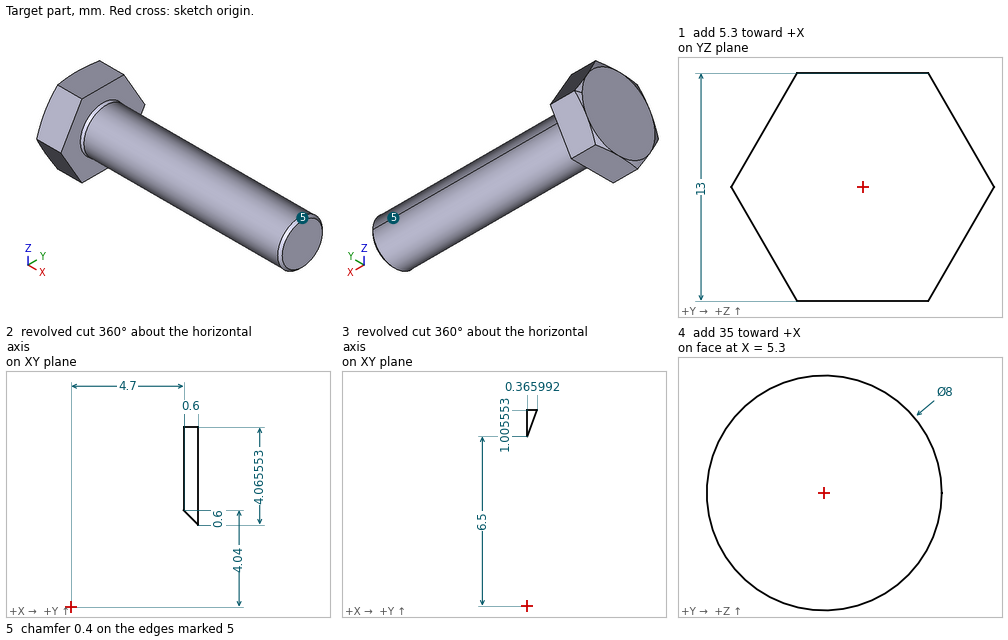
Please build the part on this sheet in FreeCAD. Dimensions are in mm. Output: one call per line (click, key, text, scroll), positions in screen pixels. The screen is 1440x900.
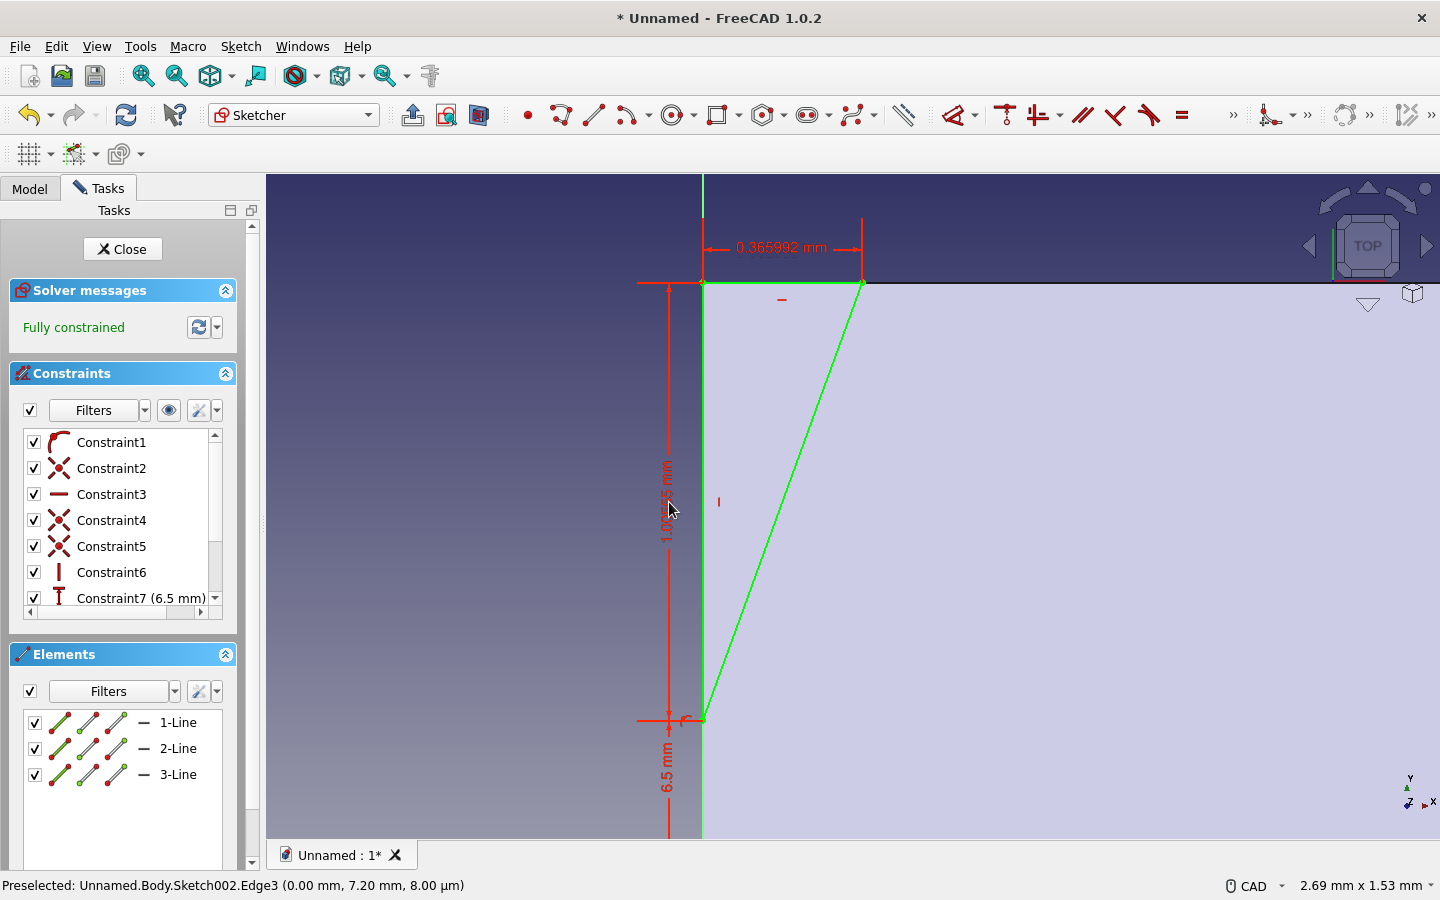
click(123, 249)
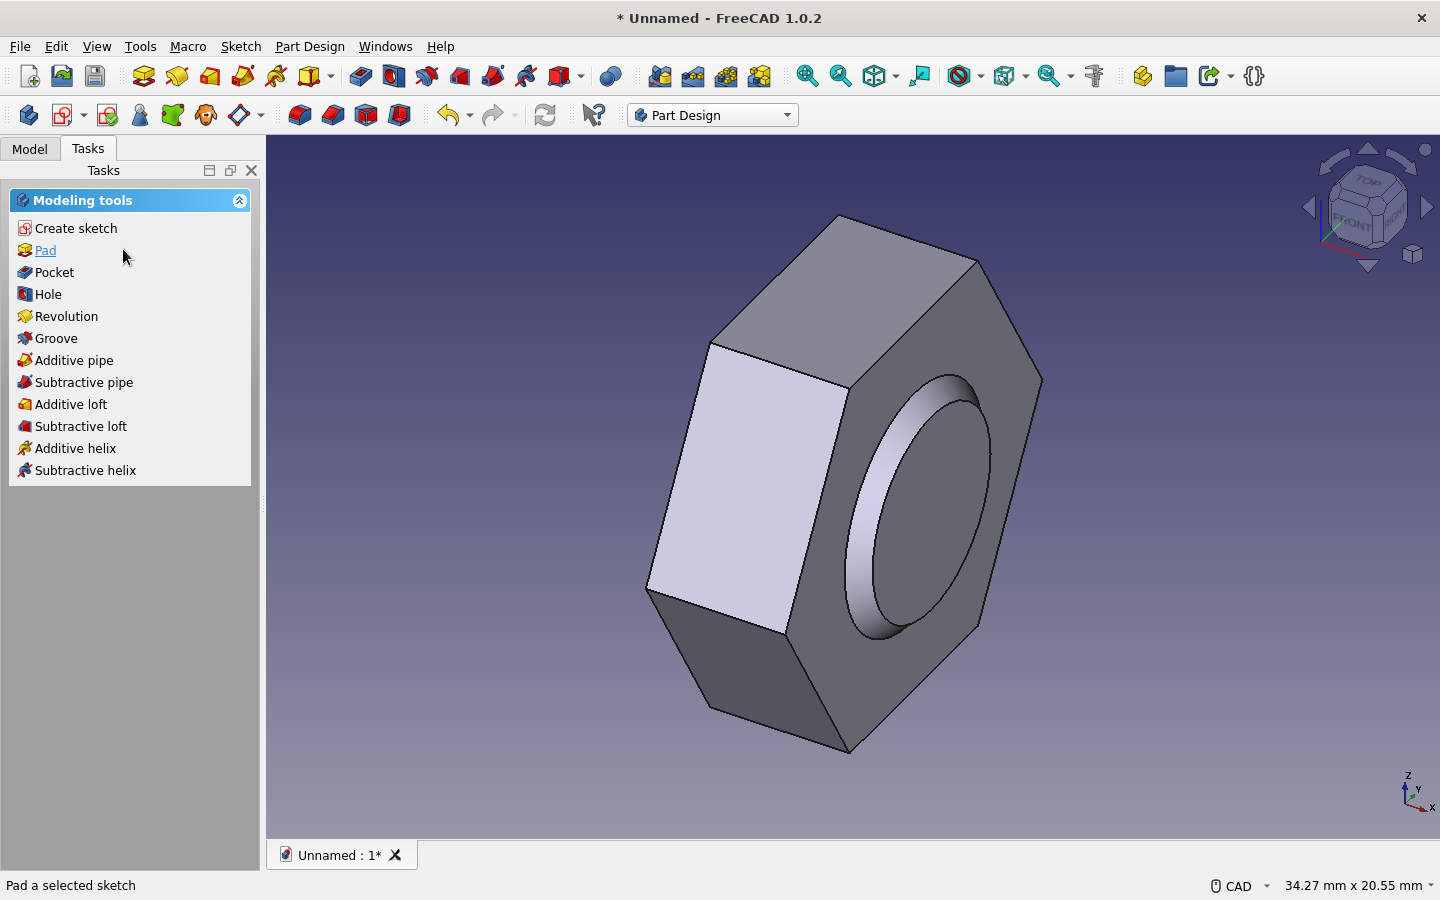
click(427, 76)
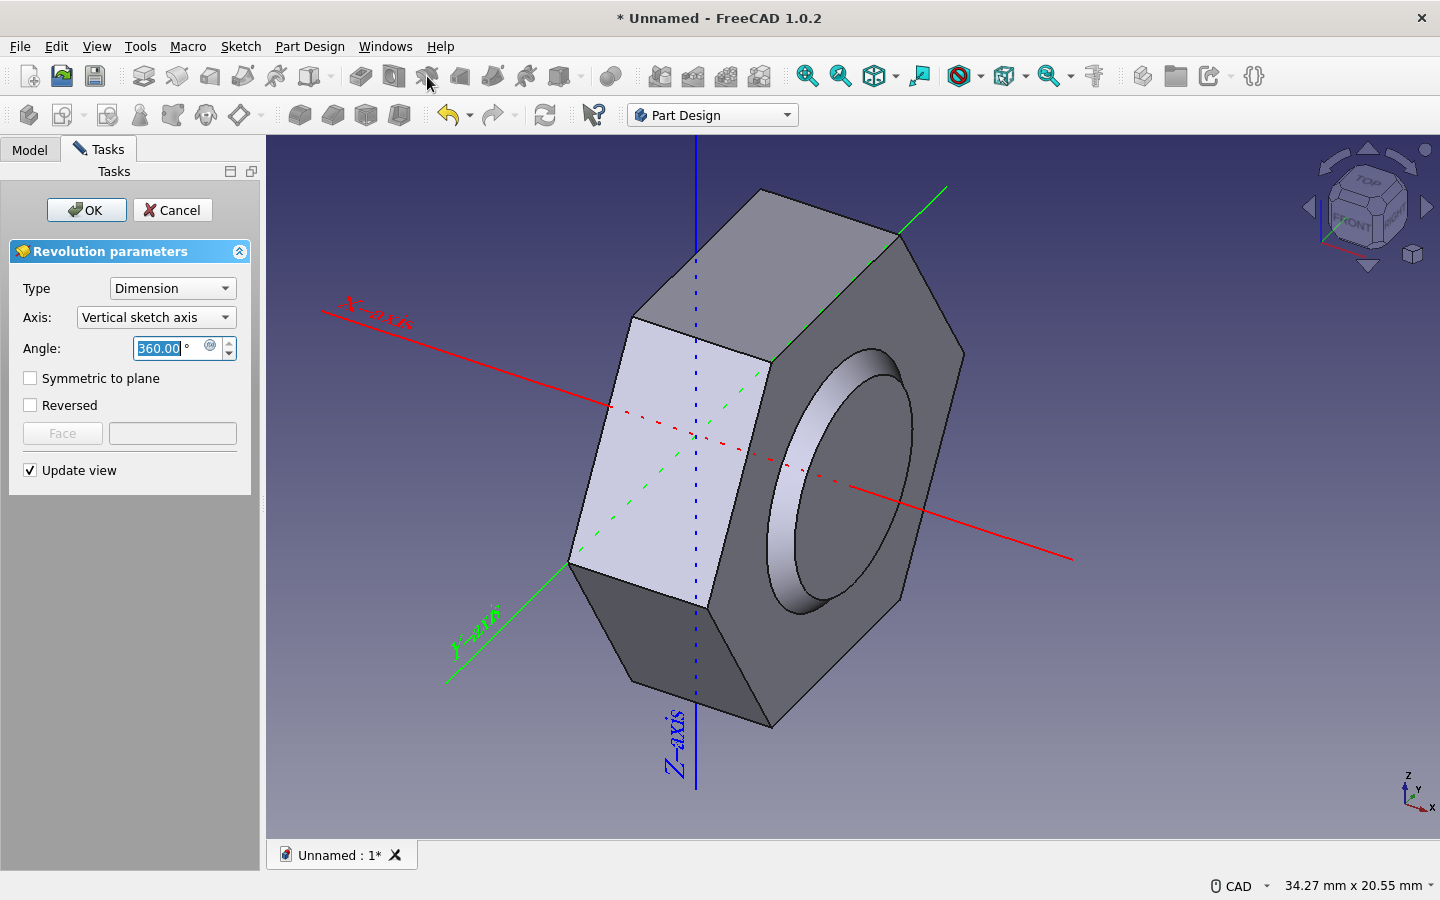
click(157, 318)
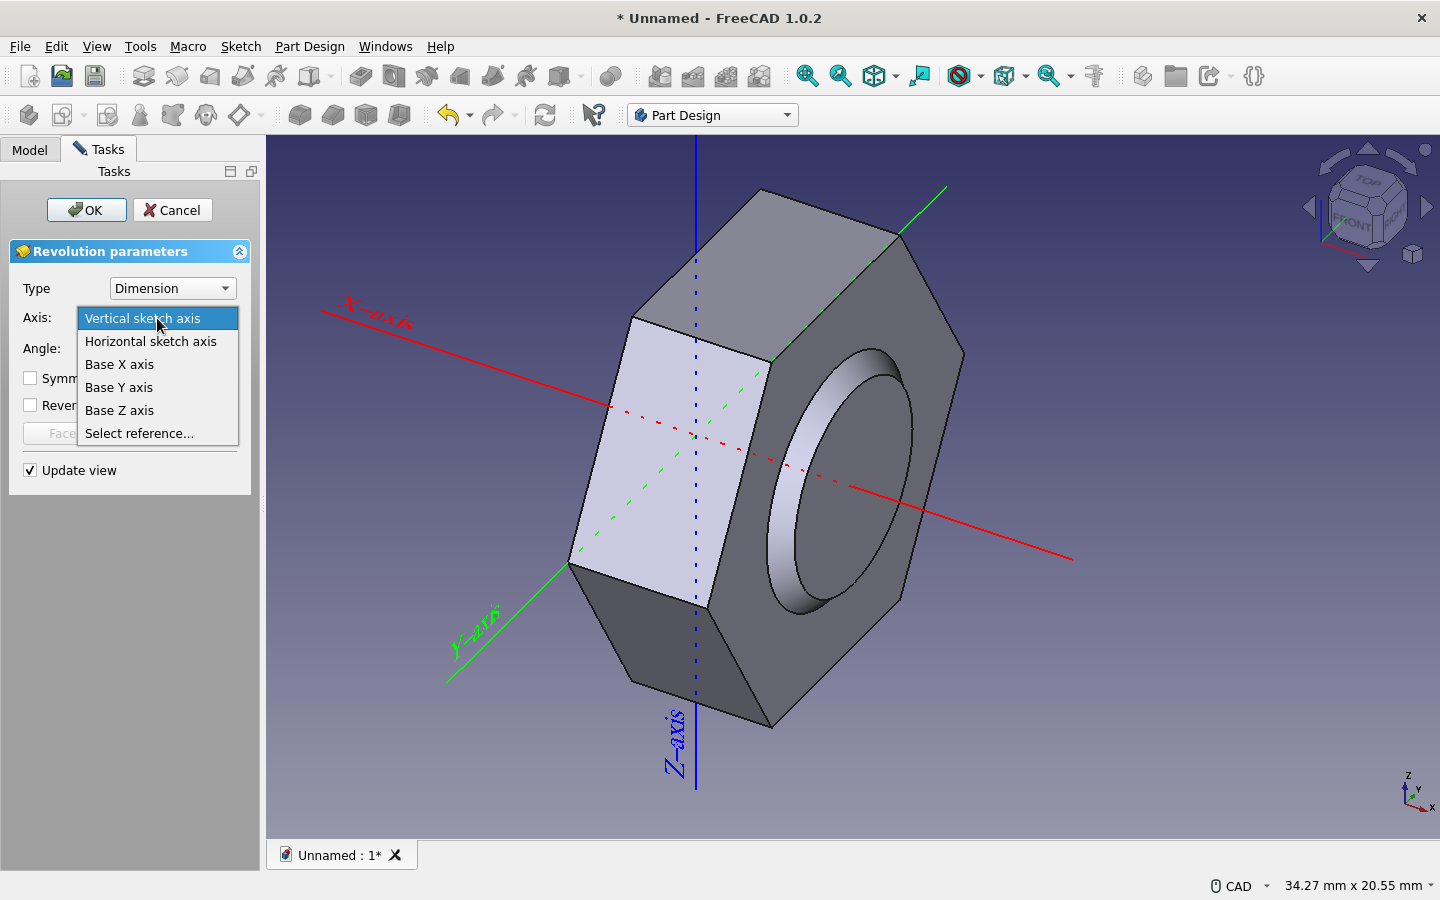
click(156, 342)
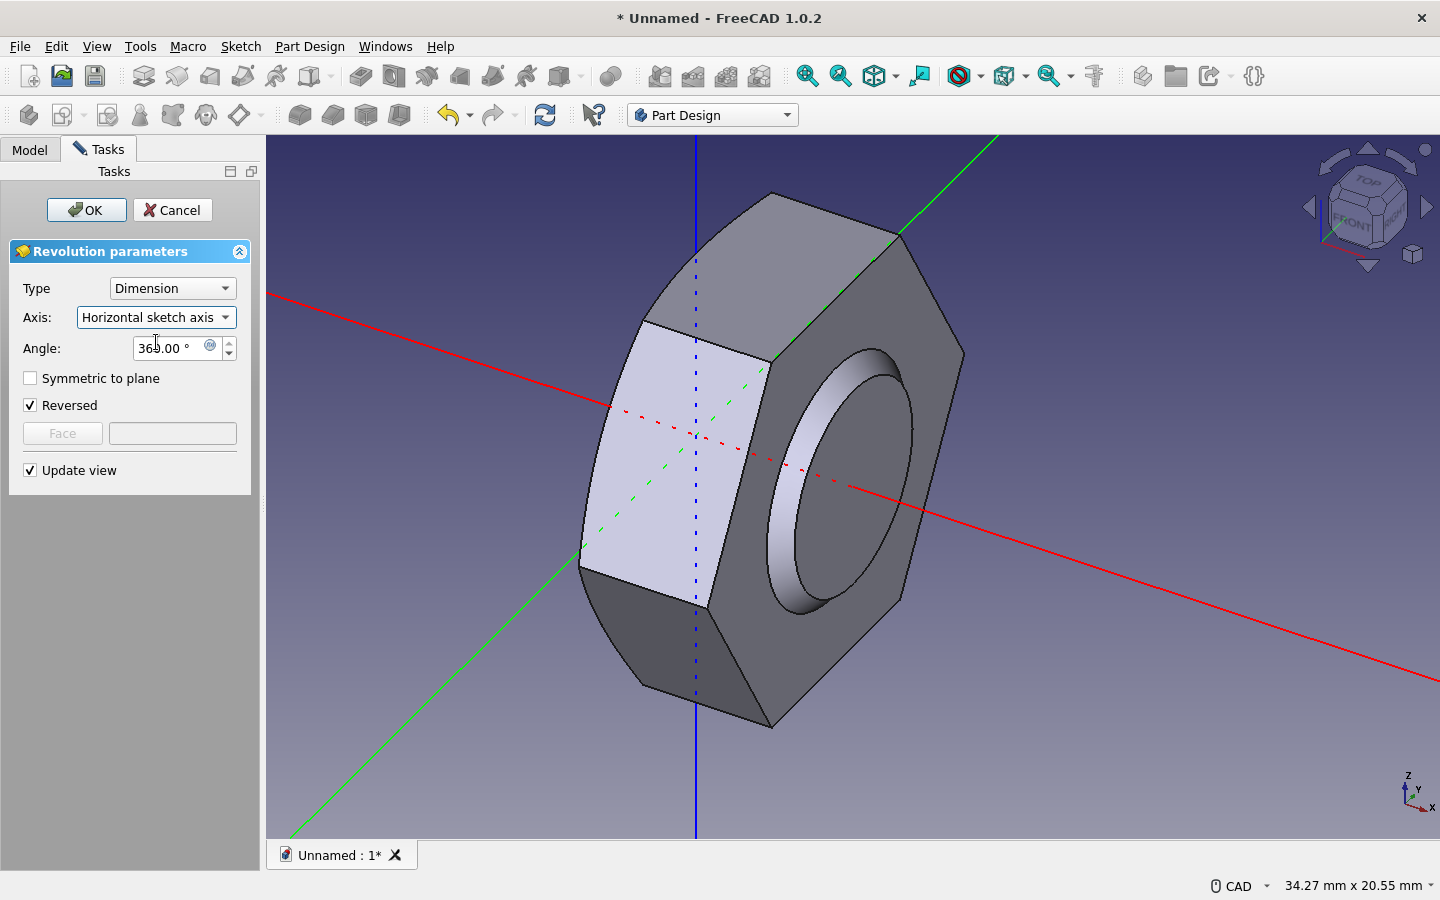
click(87, 210)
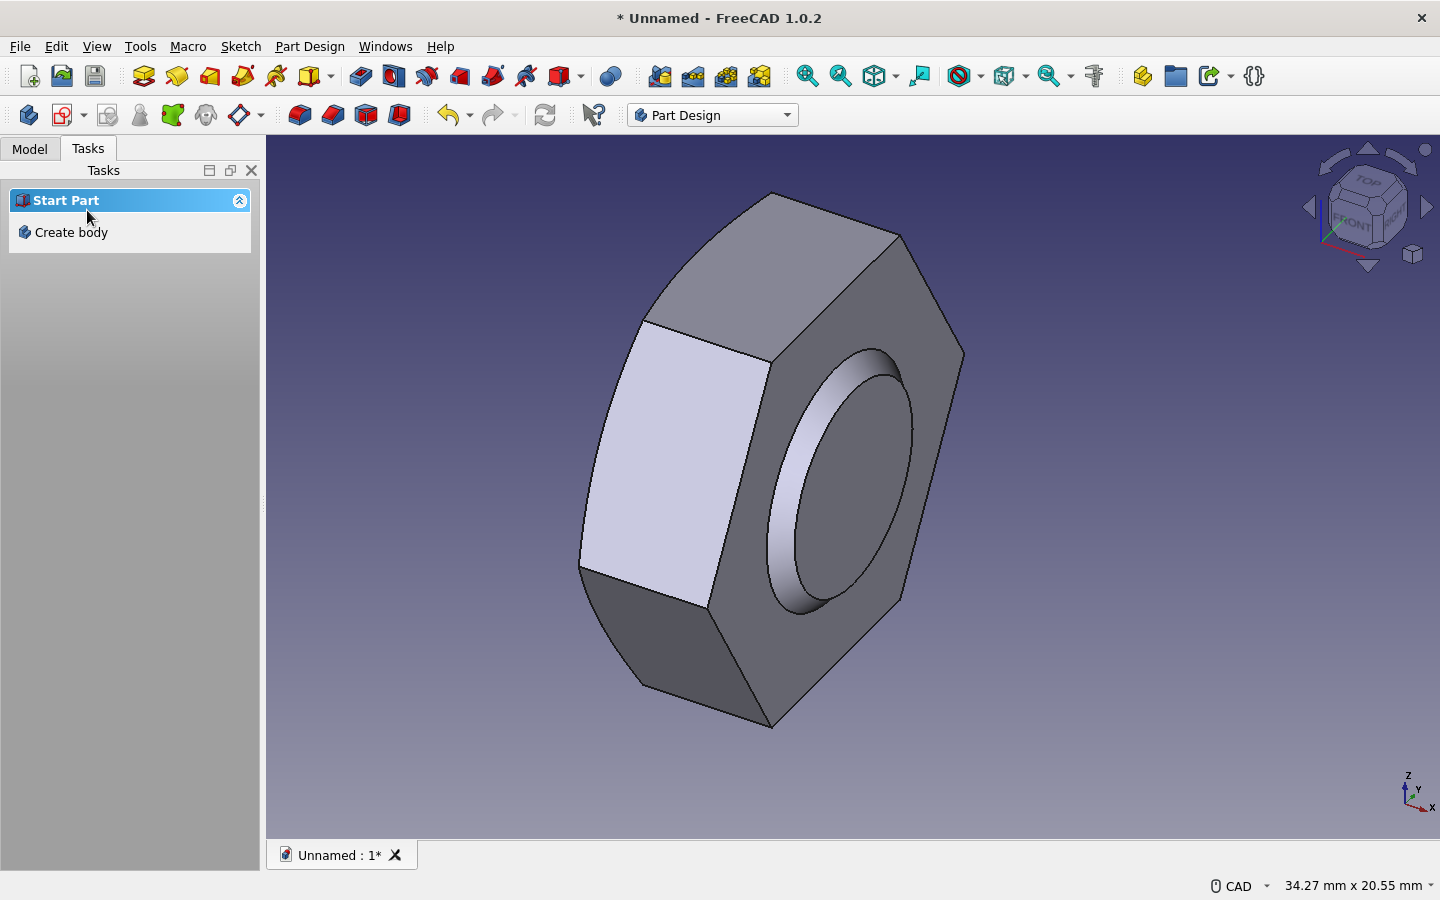
key(v)
key(f)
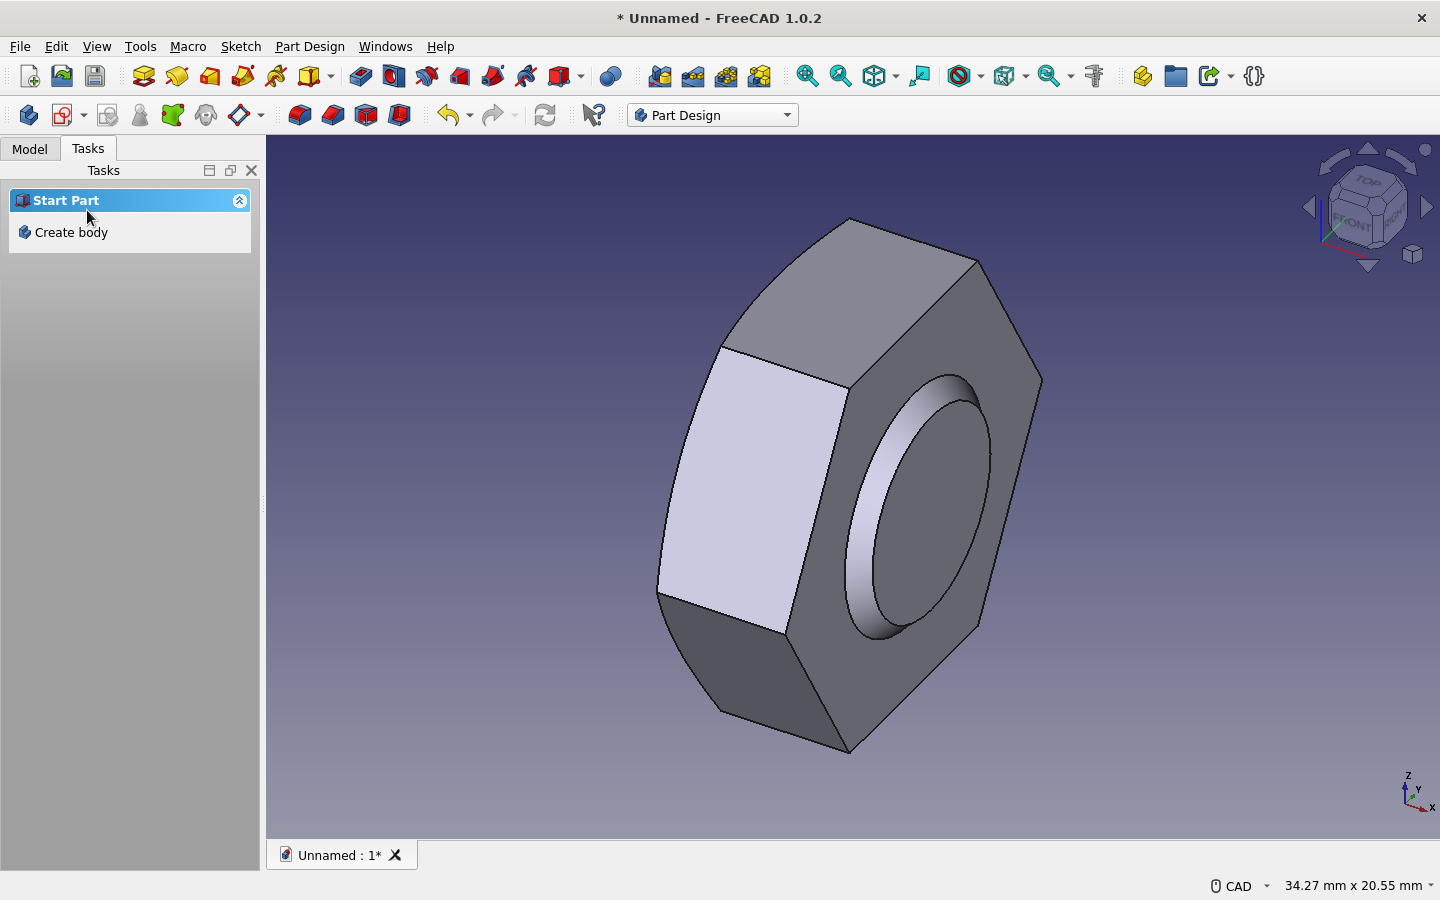
click(932, 512)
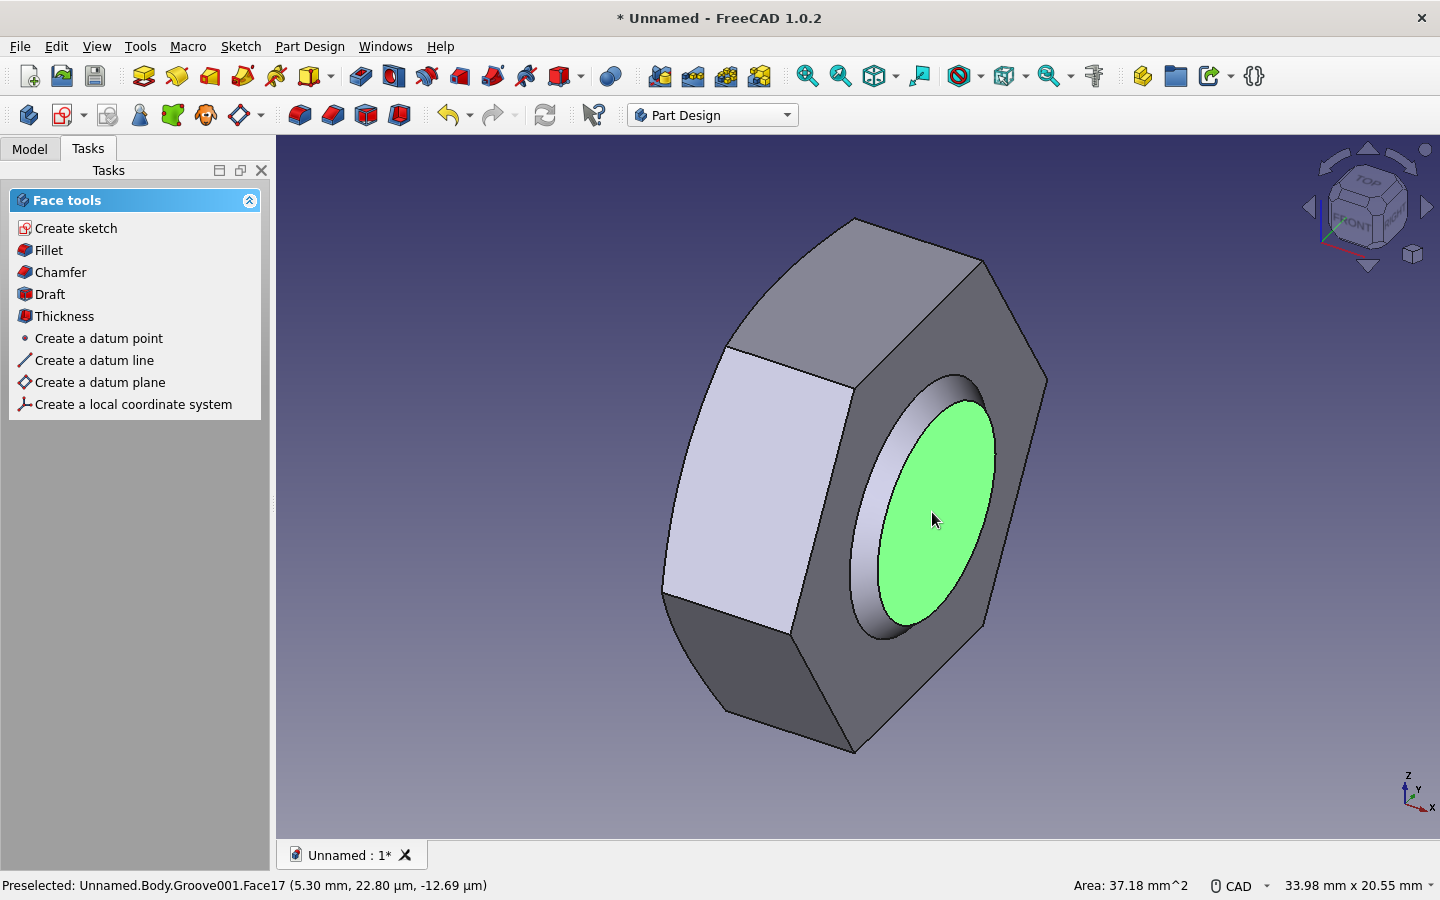
click(62, 116)